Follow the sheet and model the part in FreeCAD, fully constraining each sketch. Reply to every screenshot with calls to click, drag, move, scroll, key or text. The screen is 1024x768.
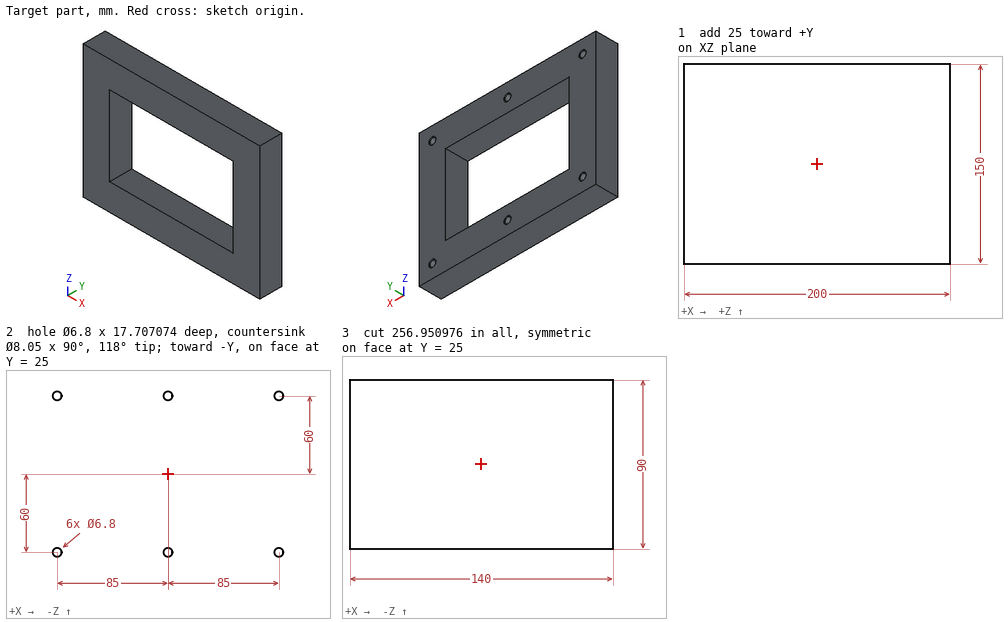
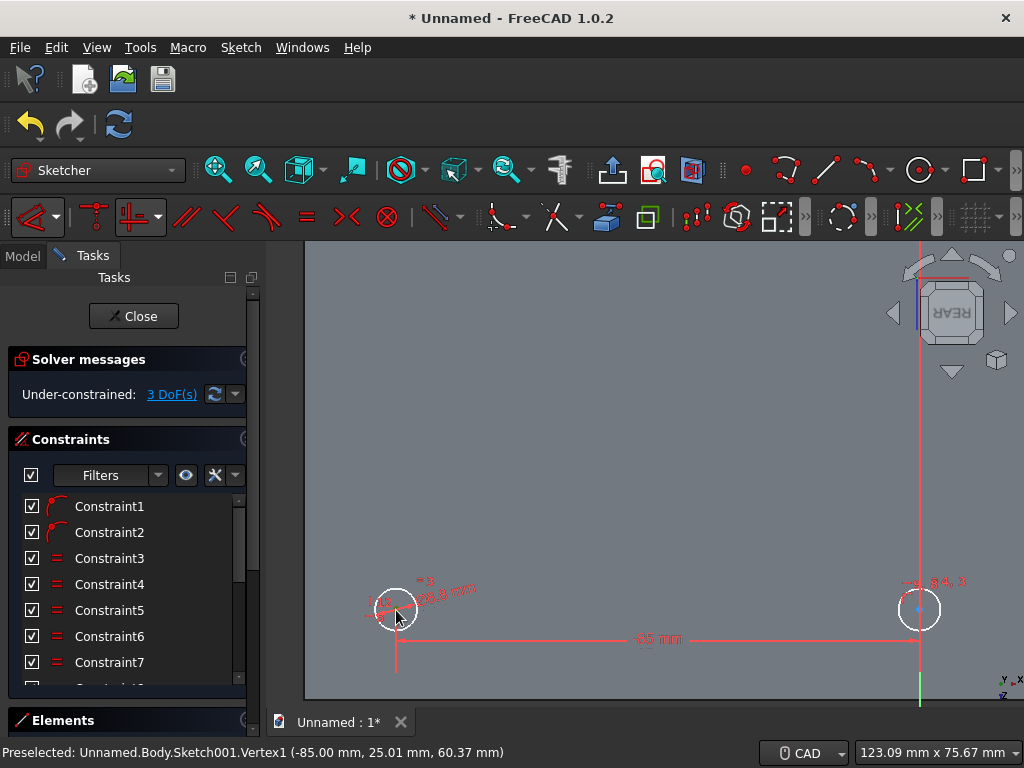
click(58, 218)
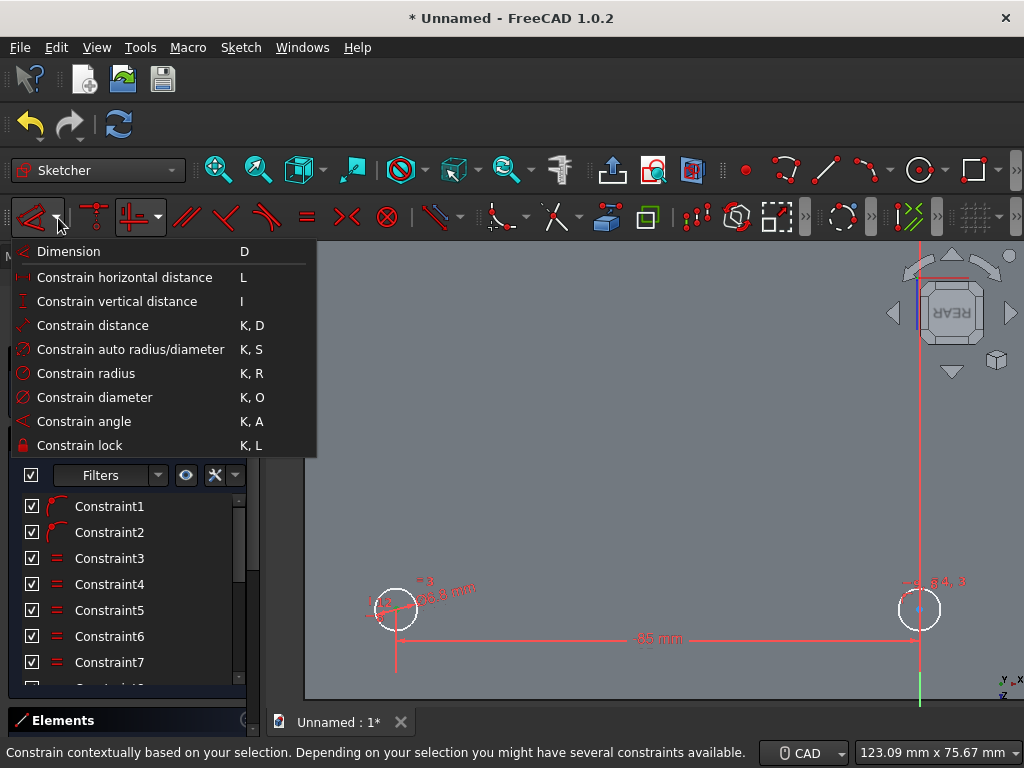
click(164, 301)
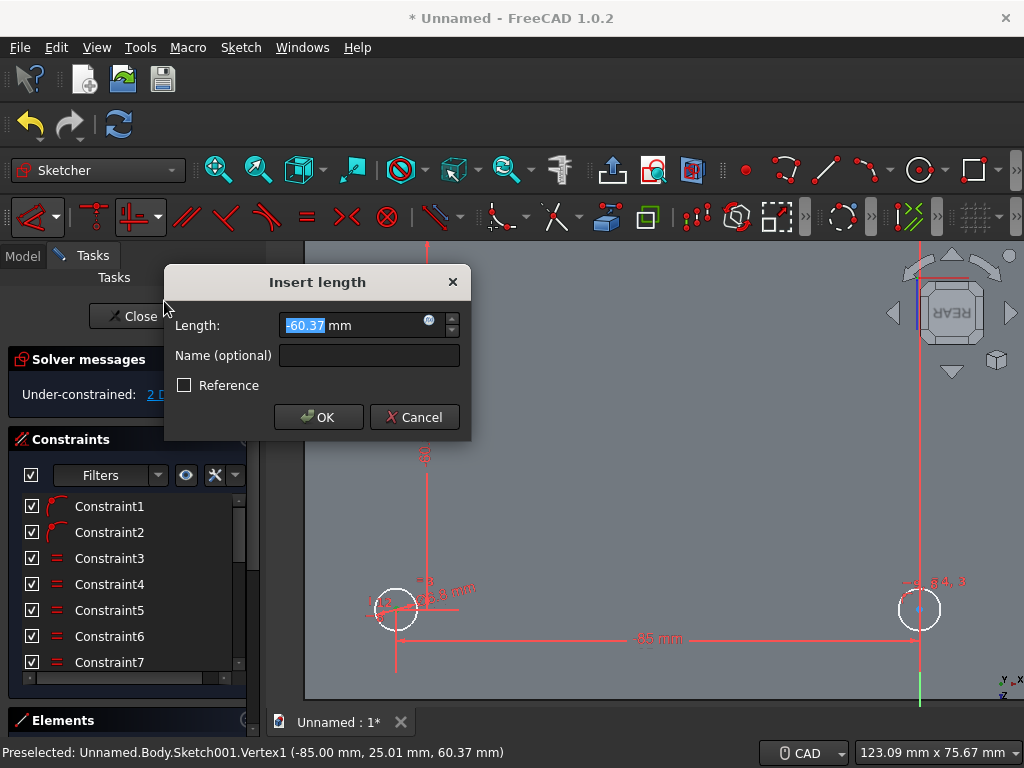
text(-60)
key(Return)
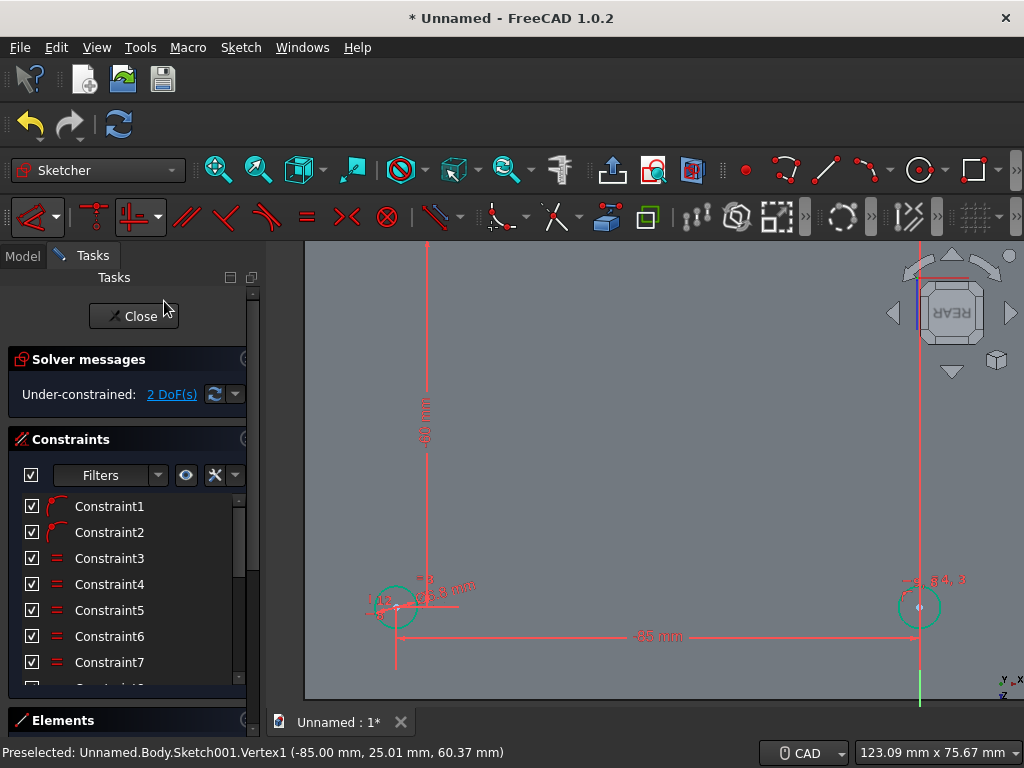
scroll(377, 611, down, 5)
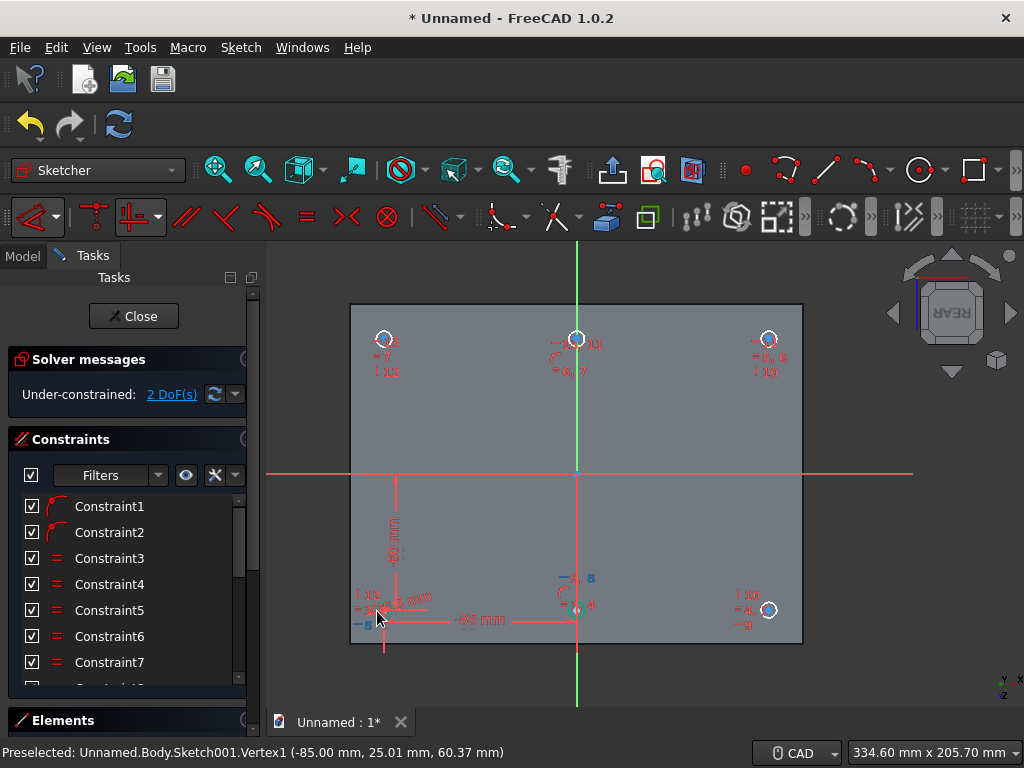
click(769, 610)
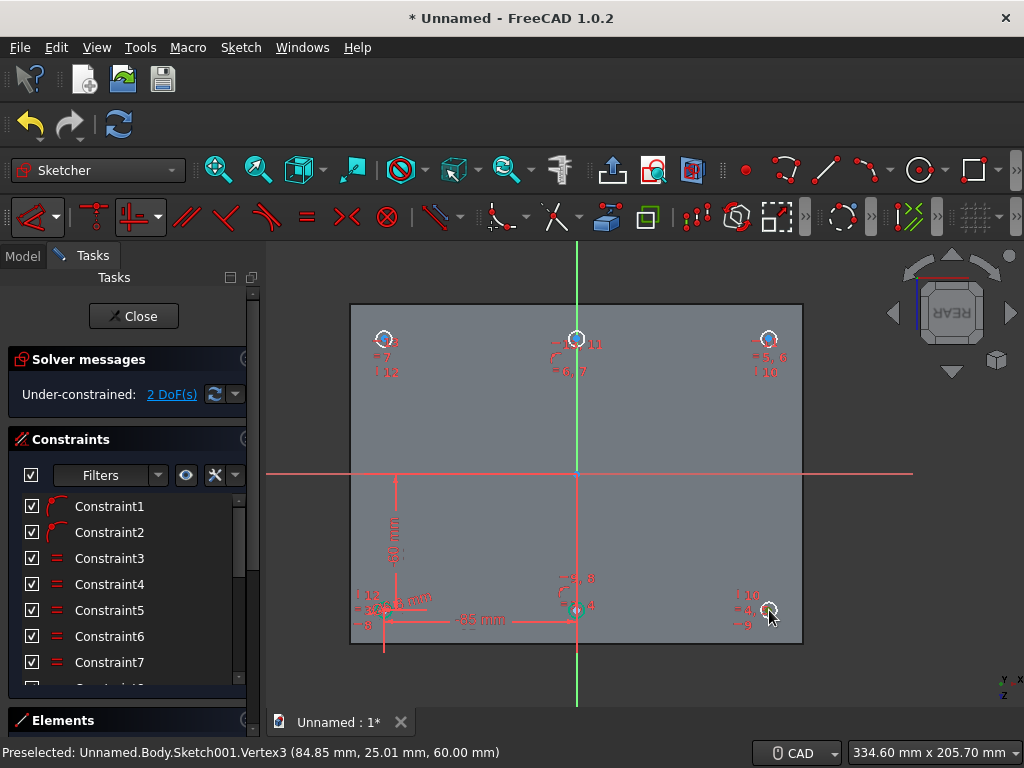
click(58, 218)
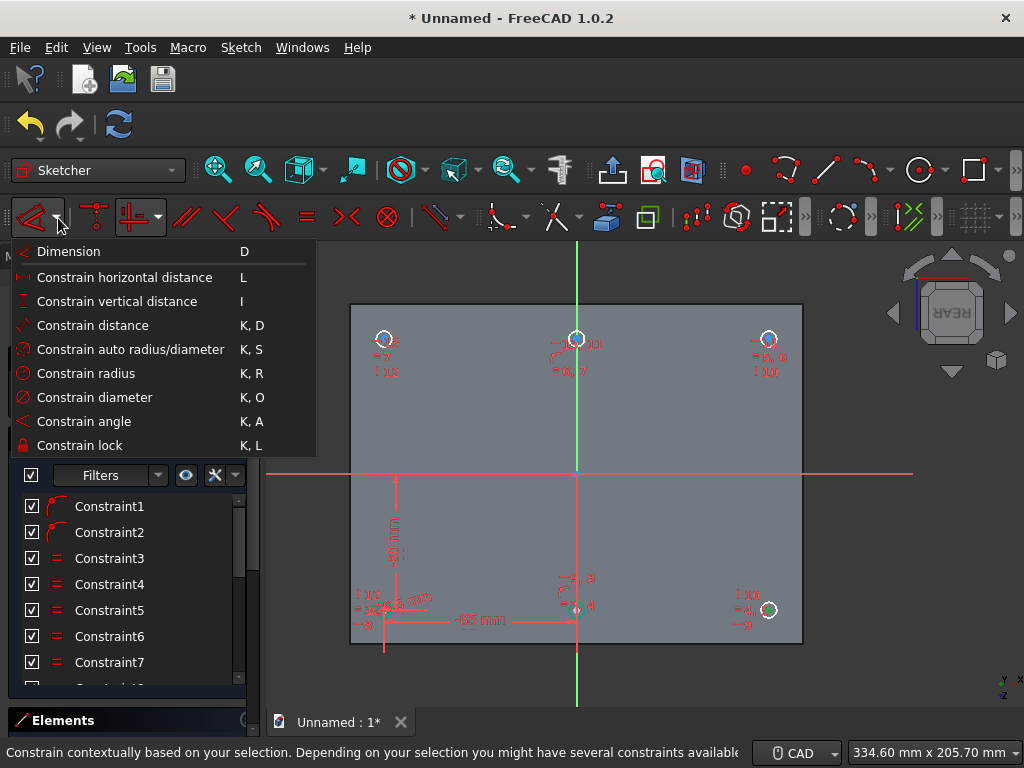
click(164, 277)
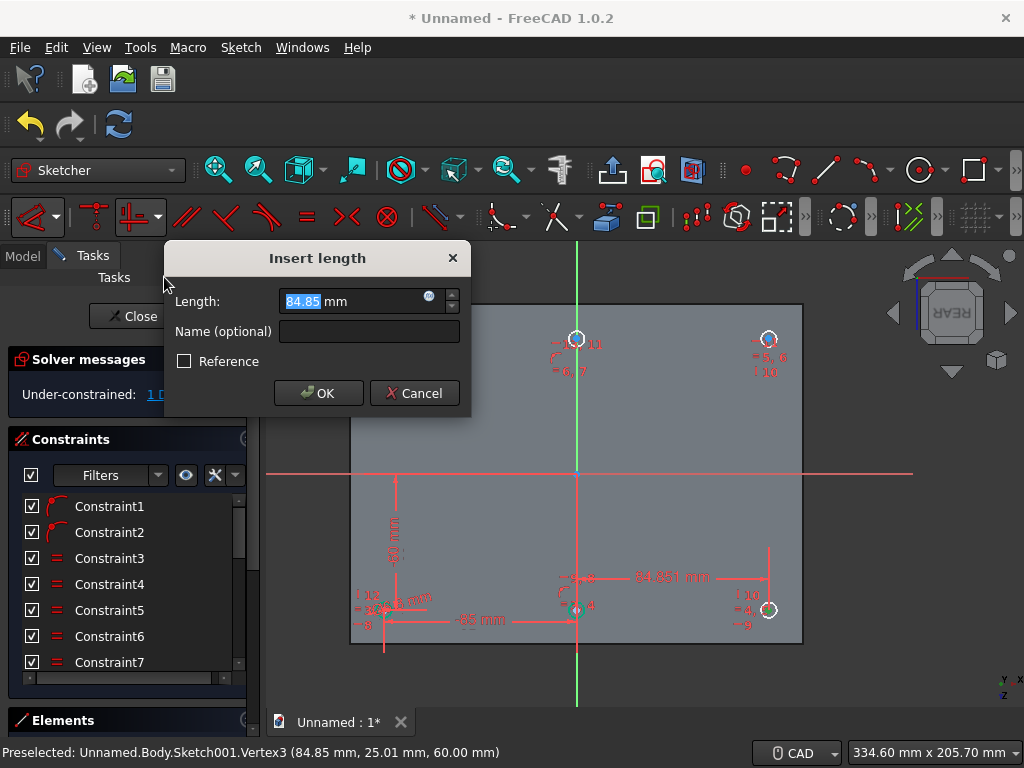
text(85)
key(Return)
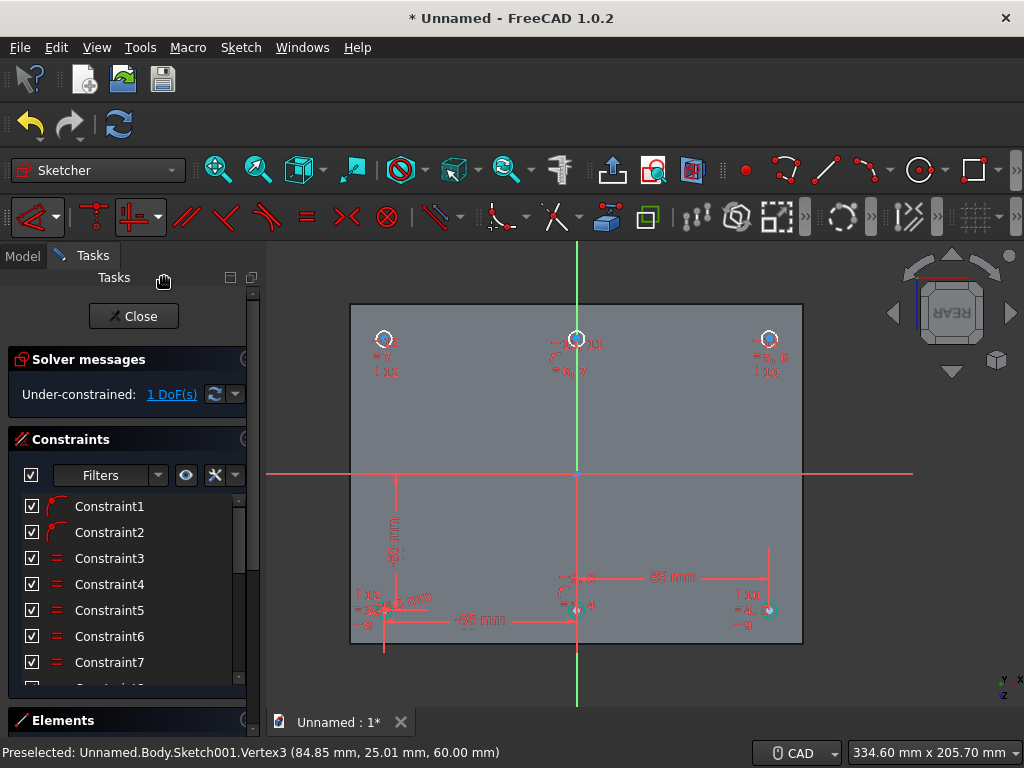
click(769, 339)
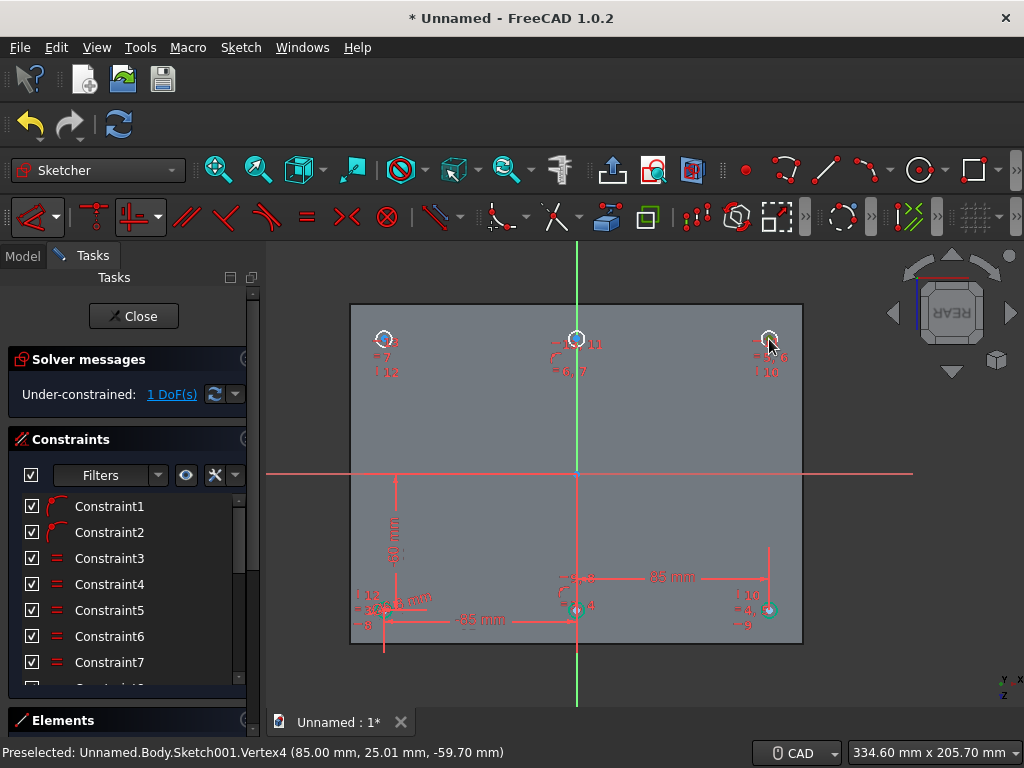
click(58, 218)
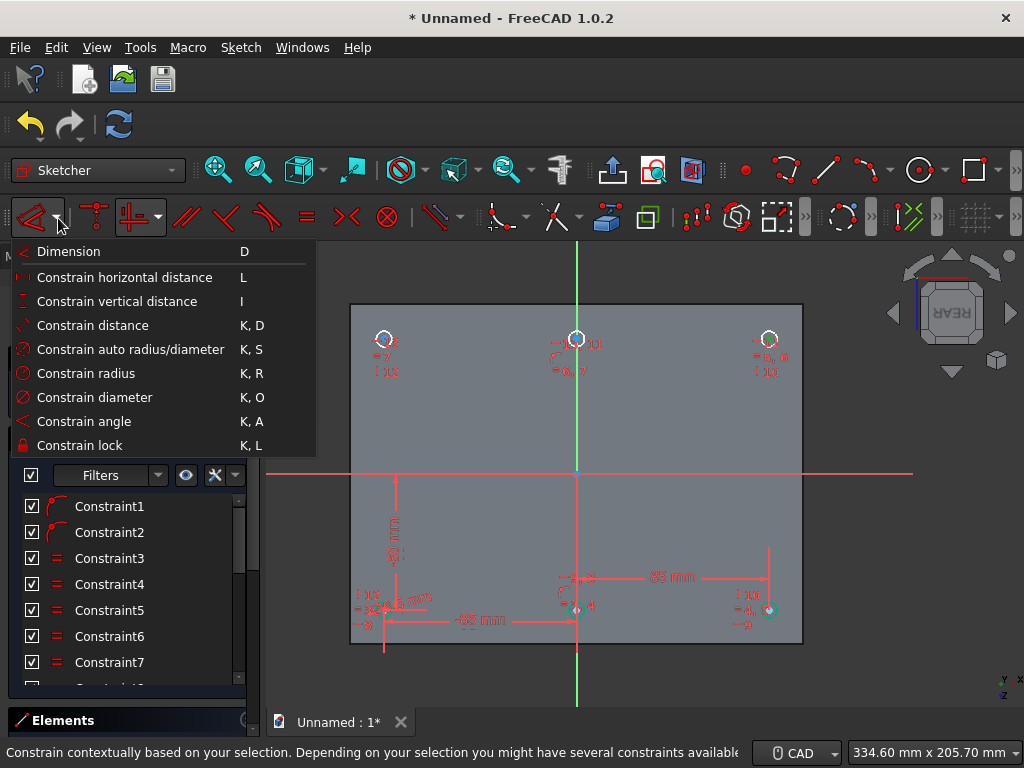
click(164, 301)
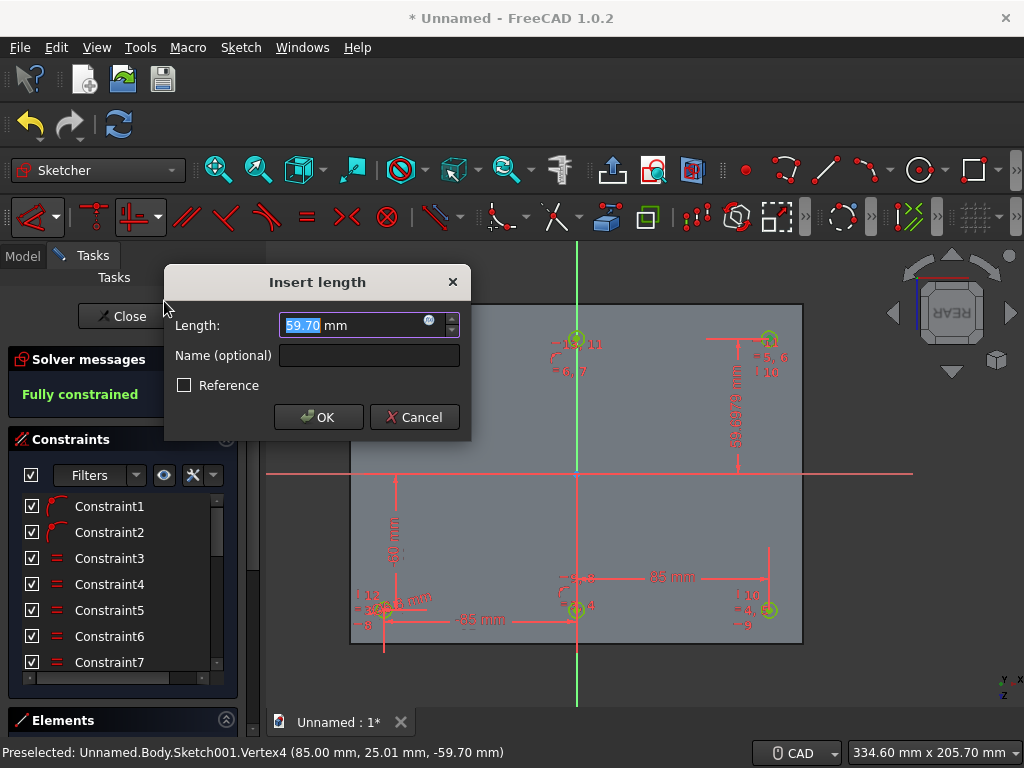
text(60)
key(Return)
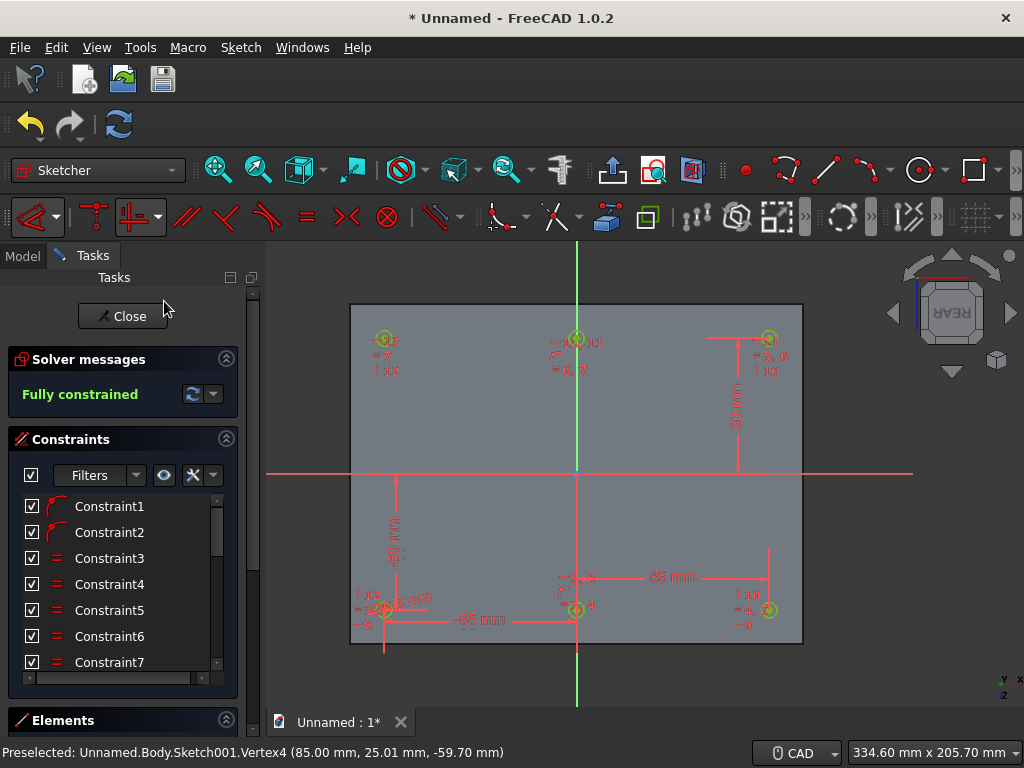
click(123, 316)